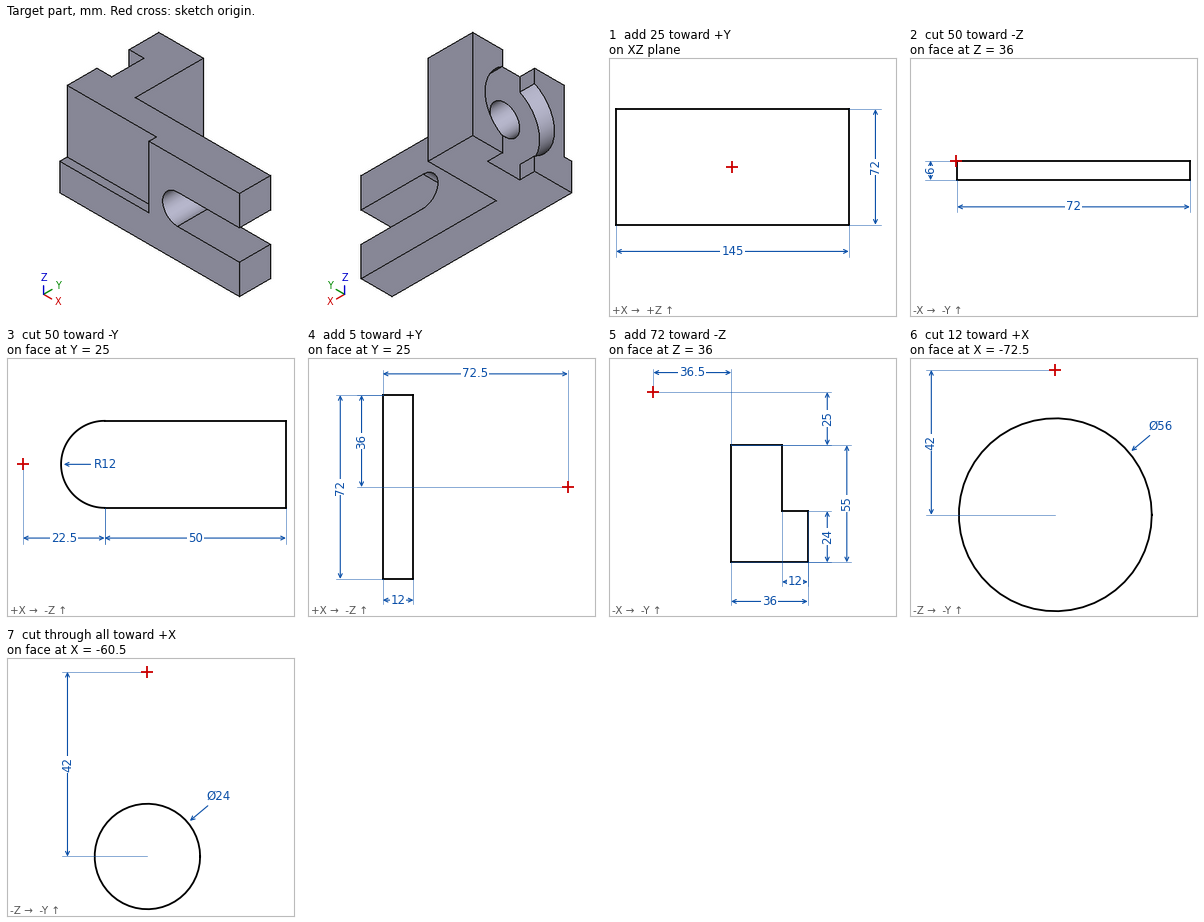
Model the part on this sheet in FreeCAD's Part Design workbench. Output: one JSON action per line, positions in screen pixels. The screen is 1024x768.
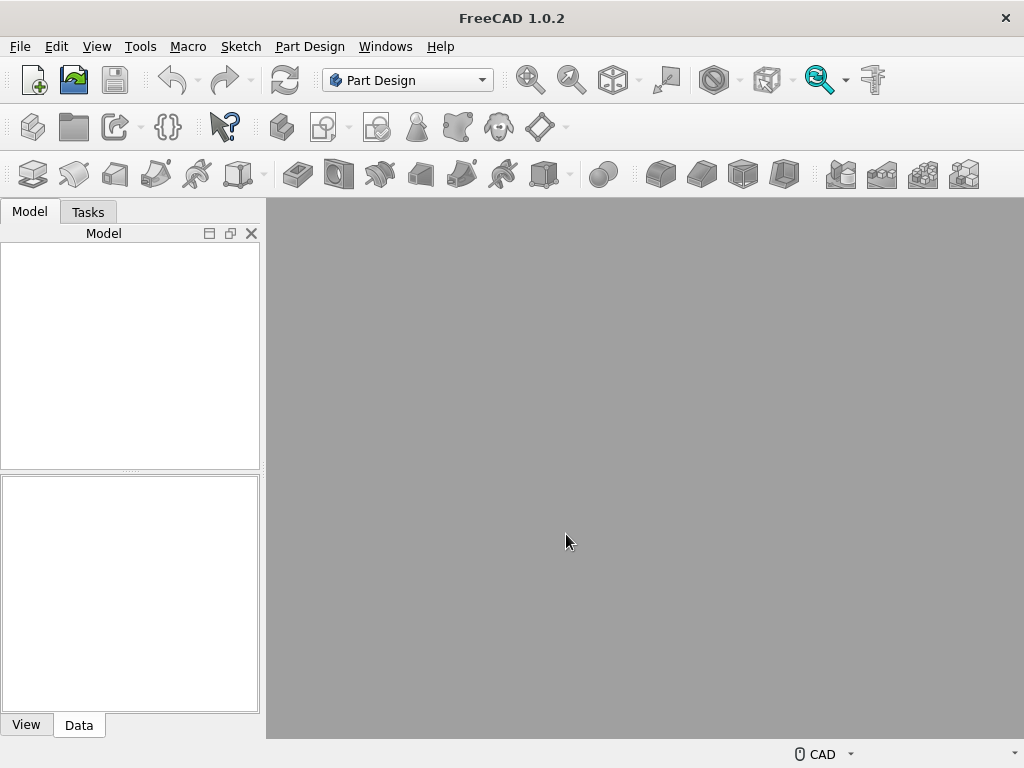
{"action": "left_click", "coordinate": [33, 80]}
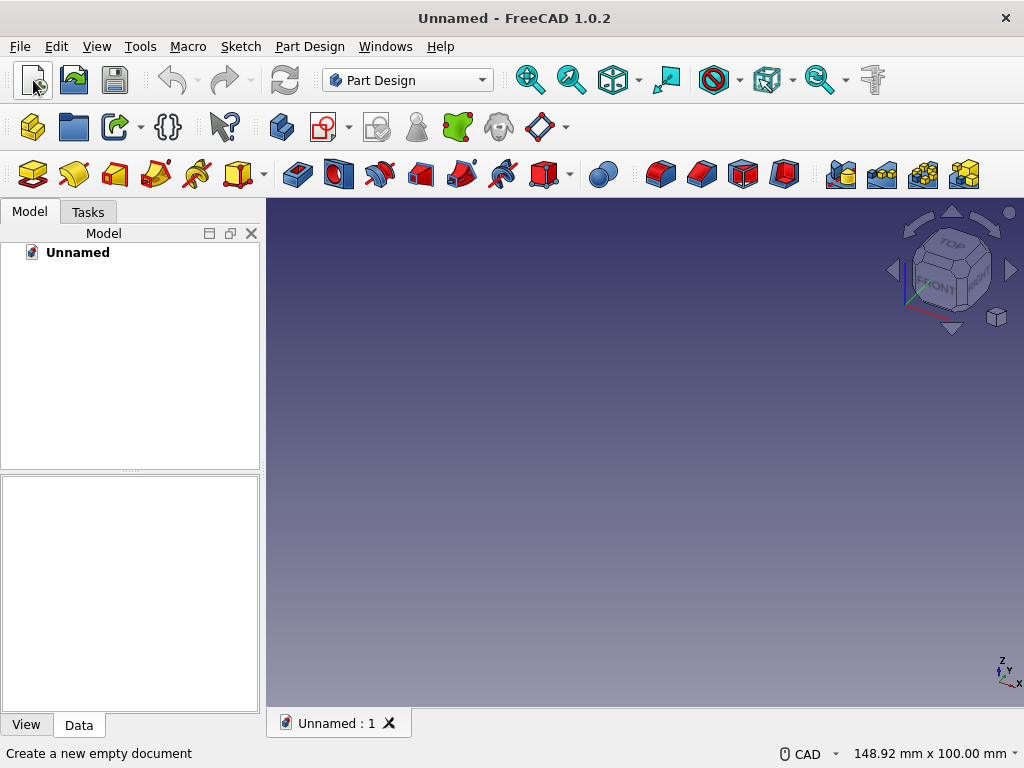
{"action": "left_click", "coordinate": [322, 128]}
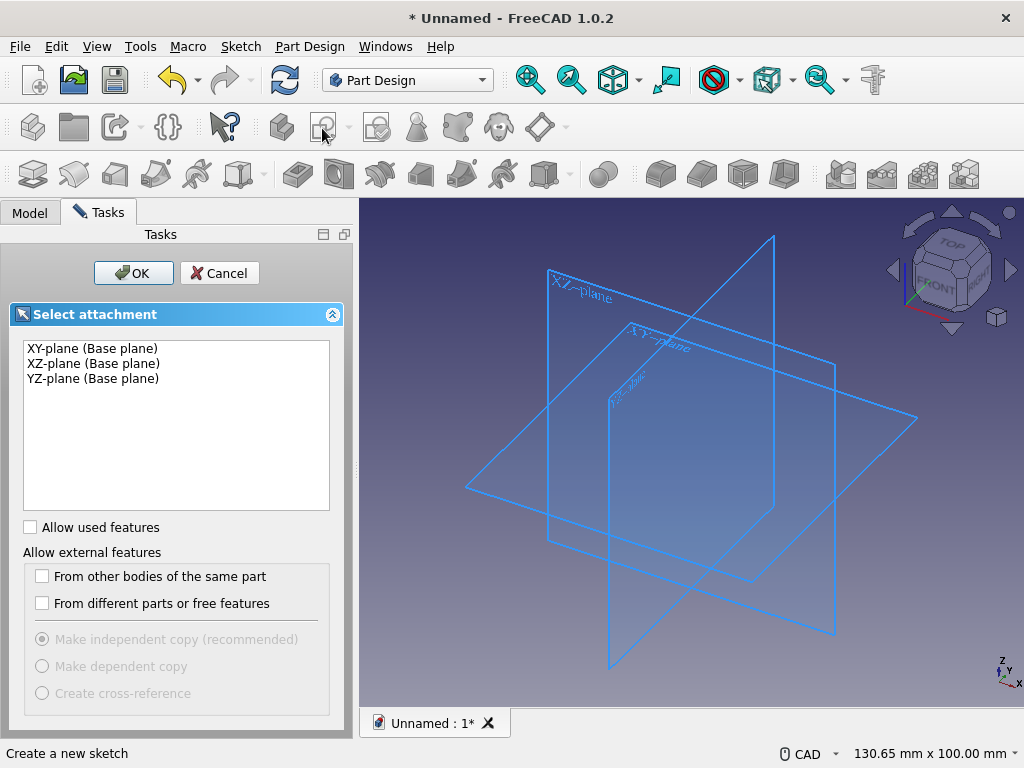
{"action": "left_click", "coordinate": [84, 364]}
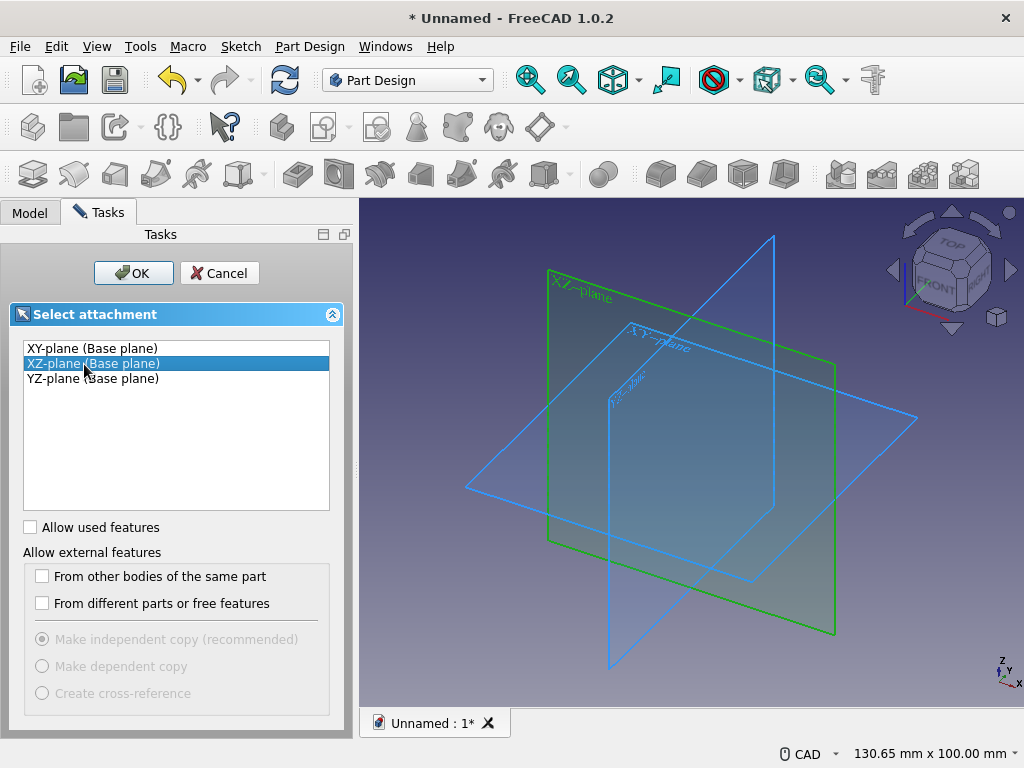
{"action": "left_click", "coordinate": [134, 273]}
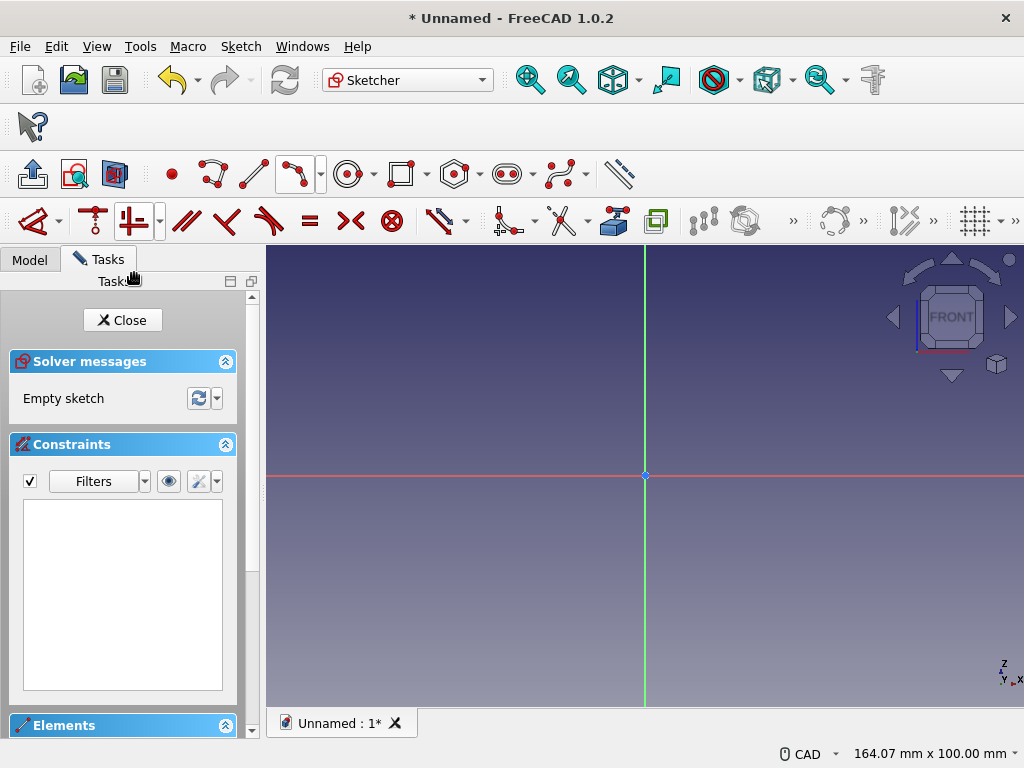
{"action": "scroll", "coordinate": [493, 476], "scroll_direction": "down", "scroll_amount": 3}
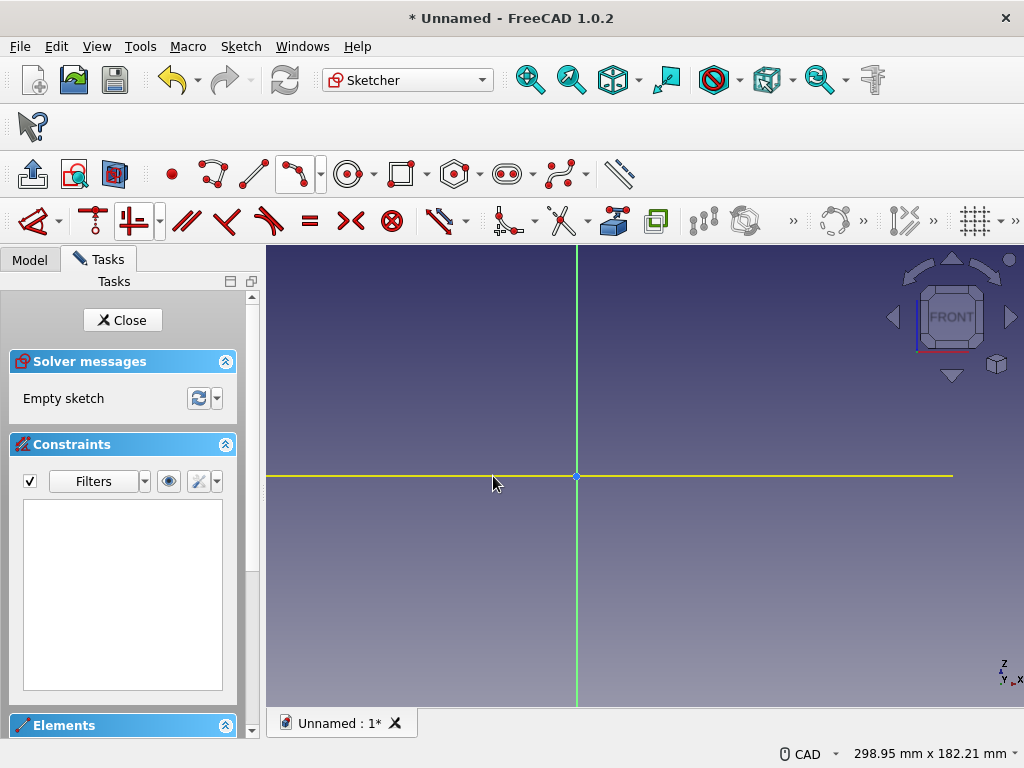
{"action": "key", "text": "g v"}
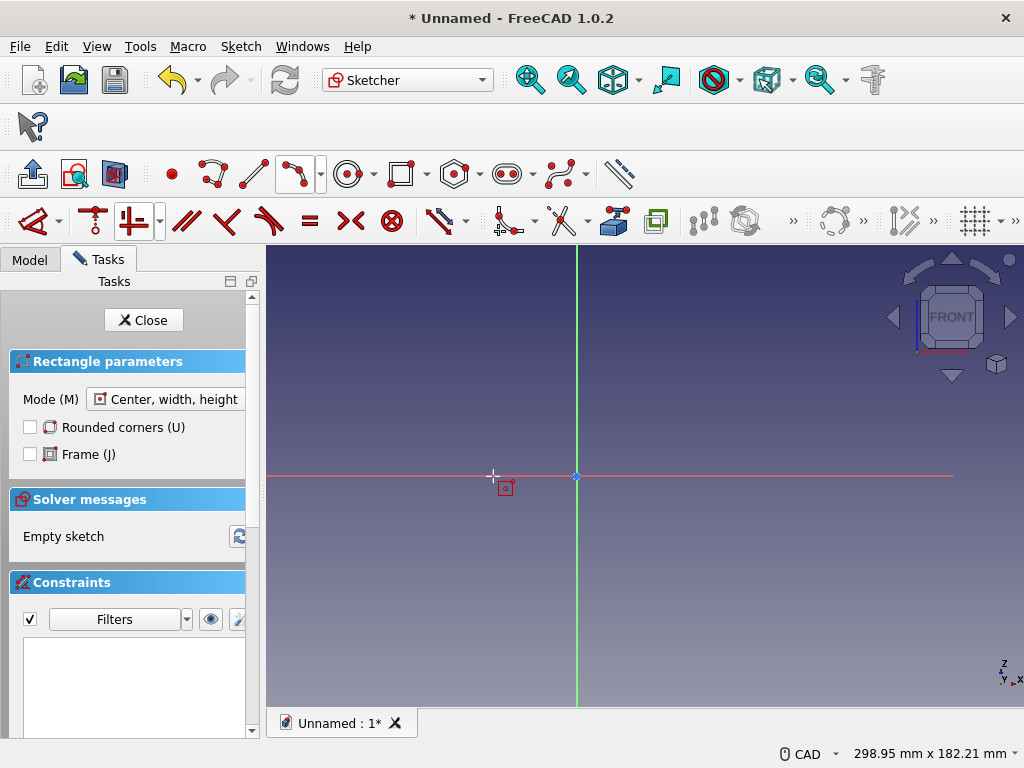
{"action": "left_click", "coordinate": [577, 476]}
{"action": "left_click", "coordinate": [760, 385]}
{"action": "key", "text": "Escape"}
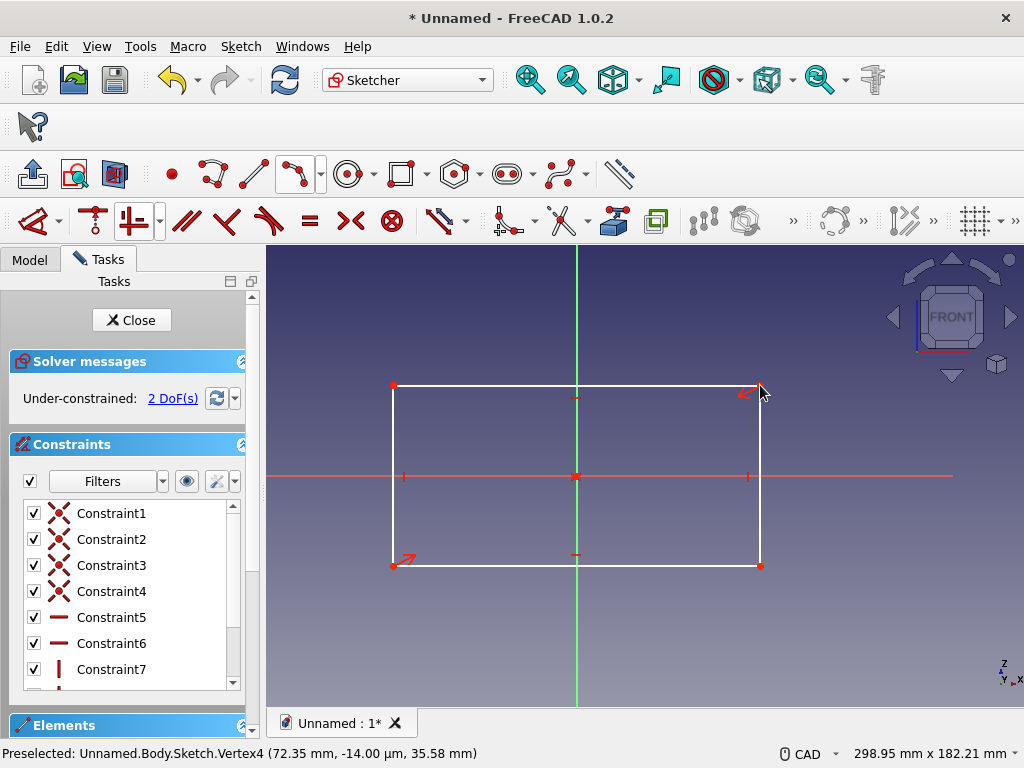
{"action": "left_click", "coordinate": [760, 512]}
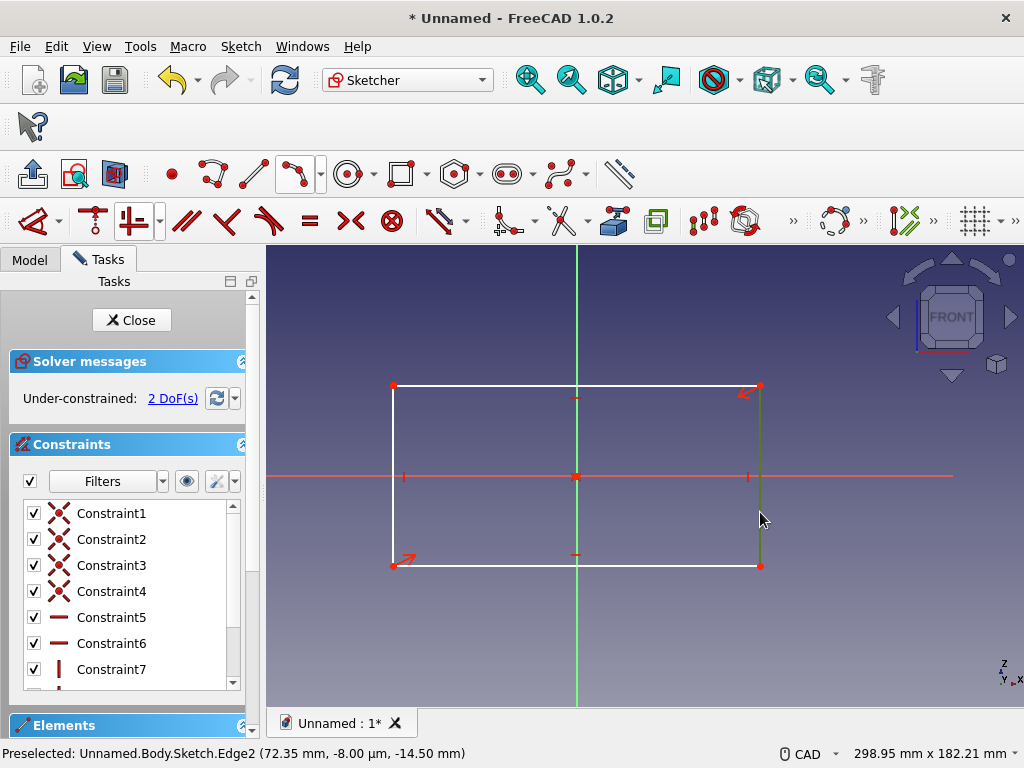
{"action": "left_click", "coordinate": [58, 222]}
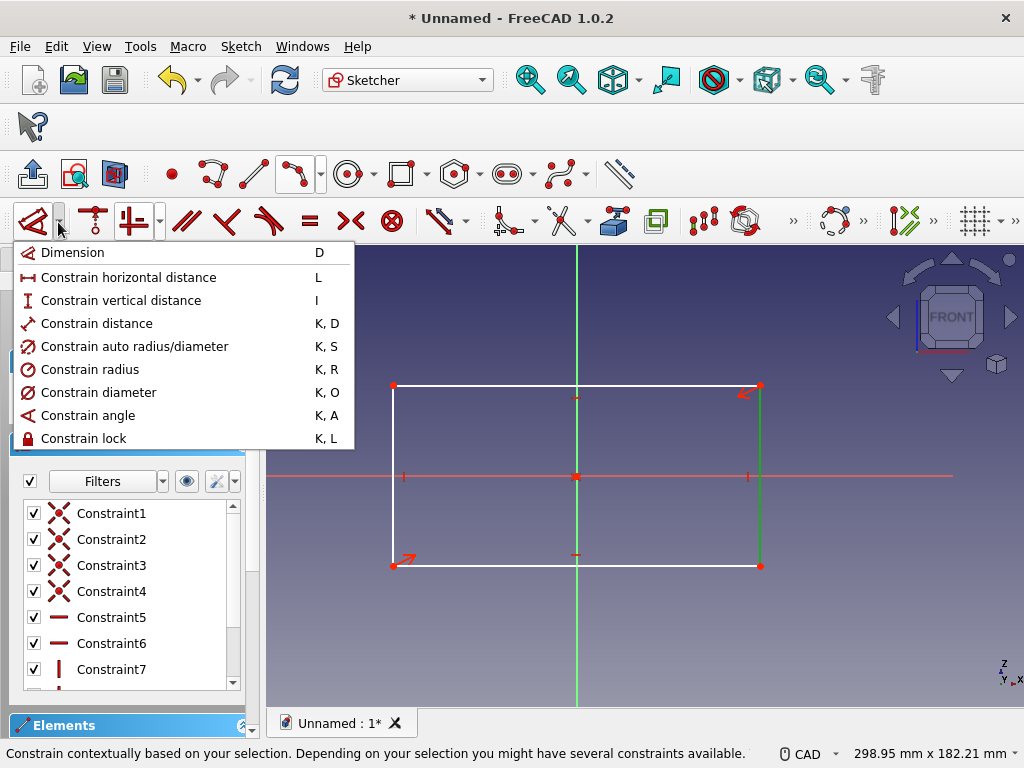
{"action": "left_click", "coordinate": [184, 300]}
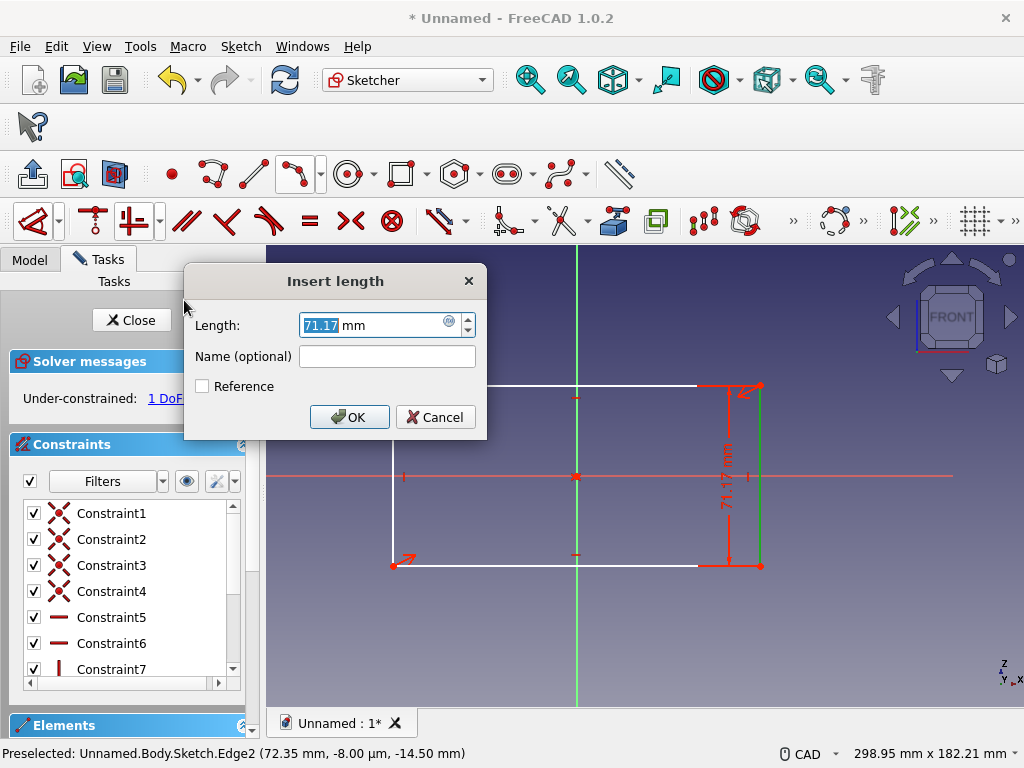
{"action": "type", "text": "72"}
{"action": "key", "text": "Return"}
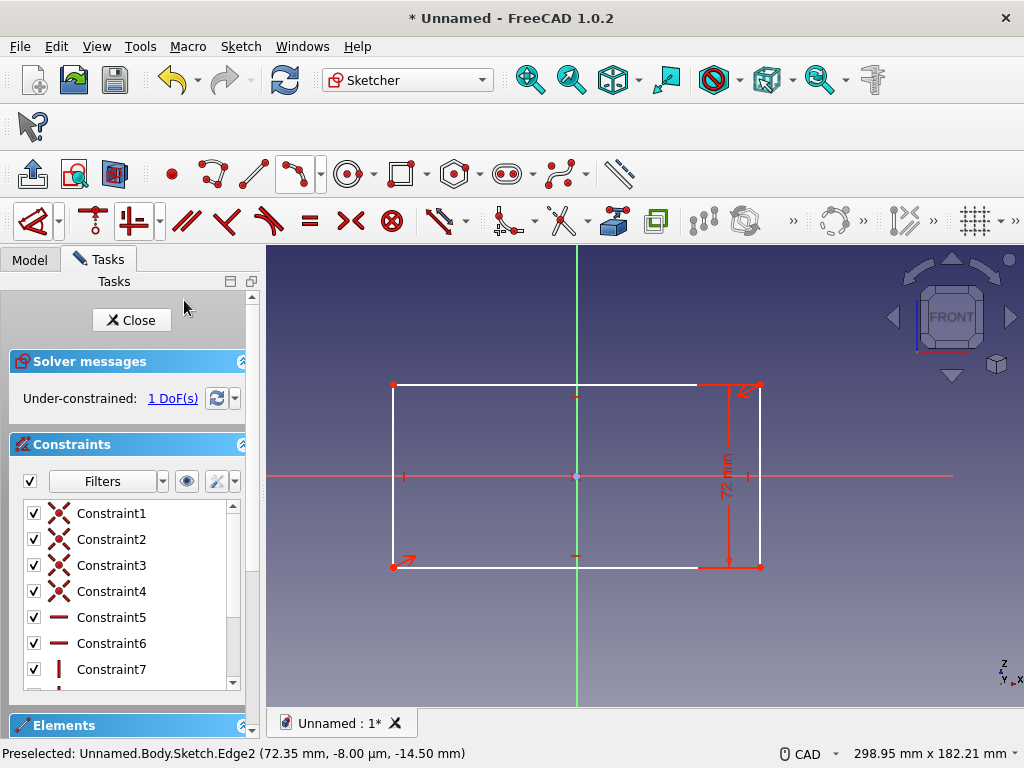
{"action": "left_click", "coordinate": [503, 568]}